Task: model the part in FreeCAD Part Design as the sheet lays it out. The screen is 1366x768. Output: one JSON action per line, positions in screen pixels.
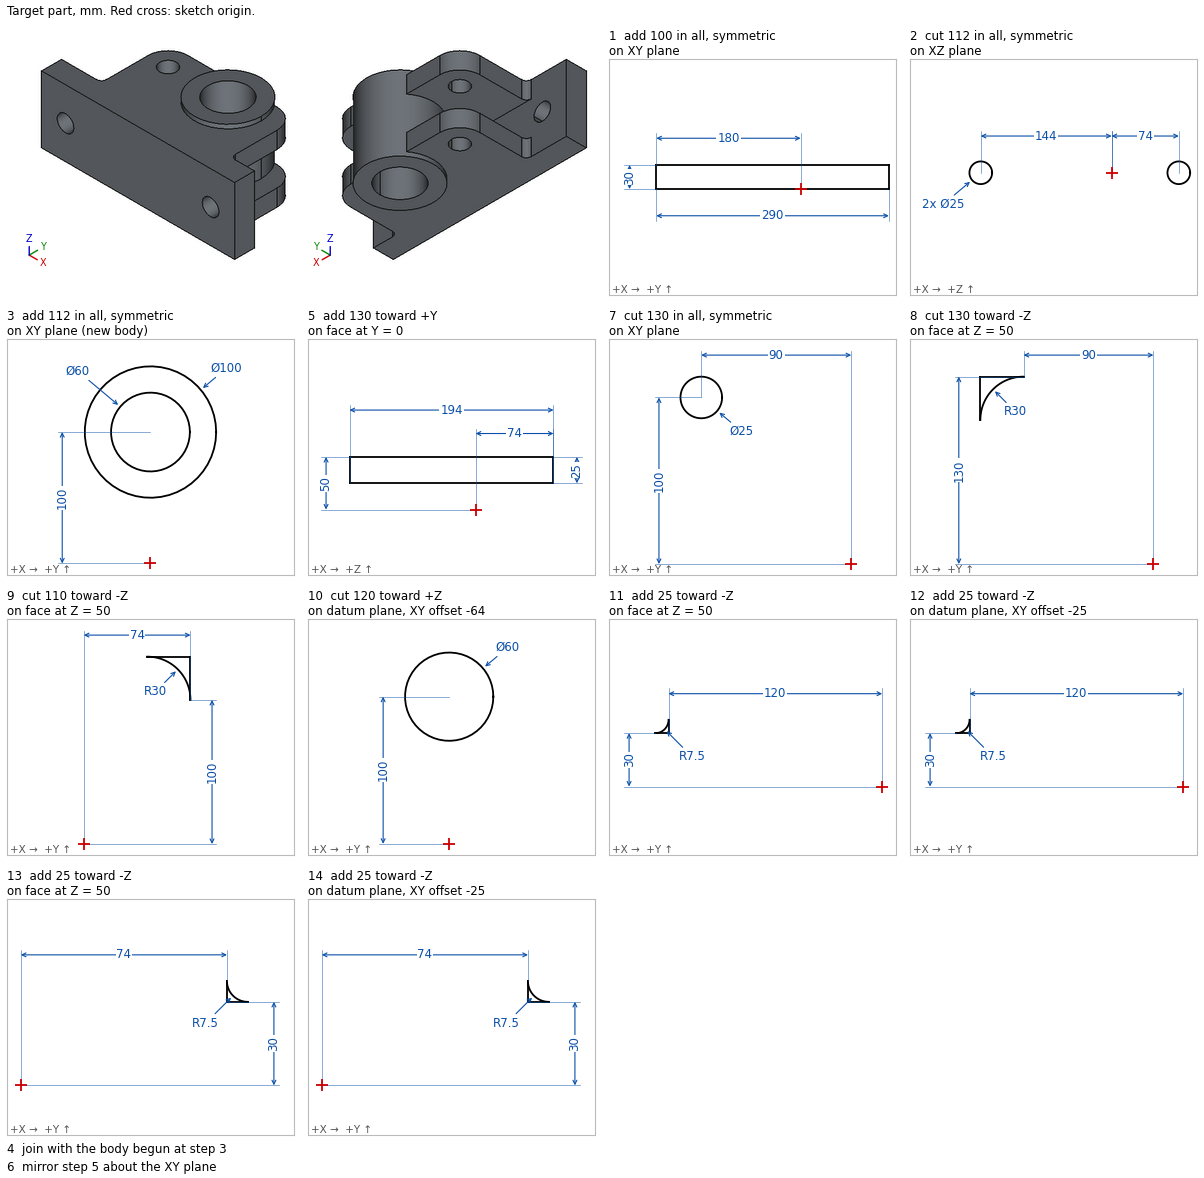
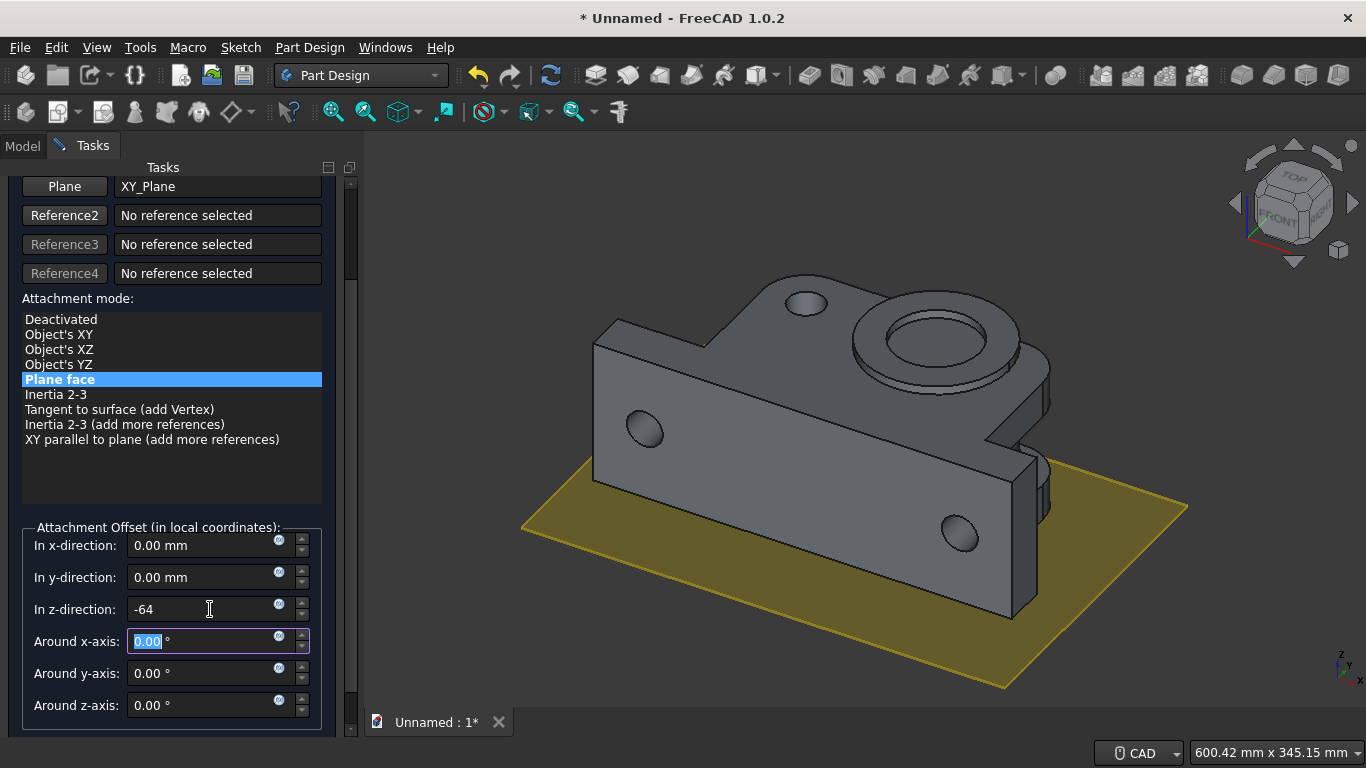
{"action": "scroll", "coordinate": [351, 456], "scroll_direction": "up", "scroll_amount": 3}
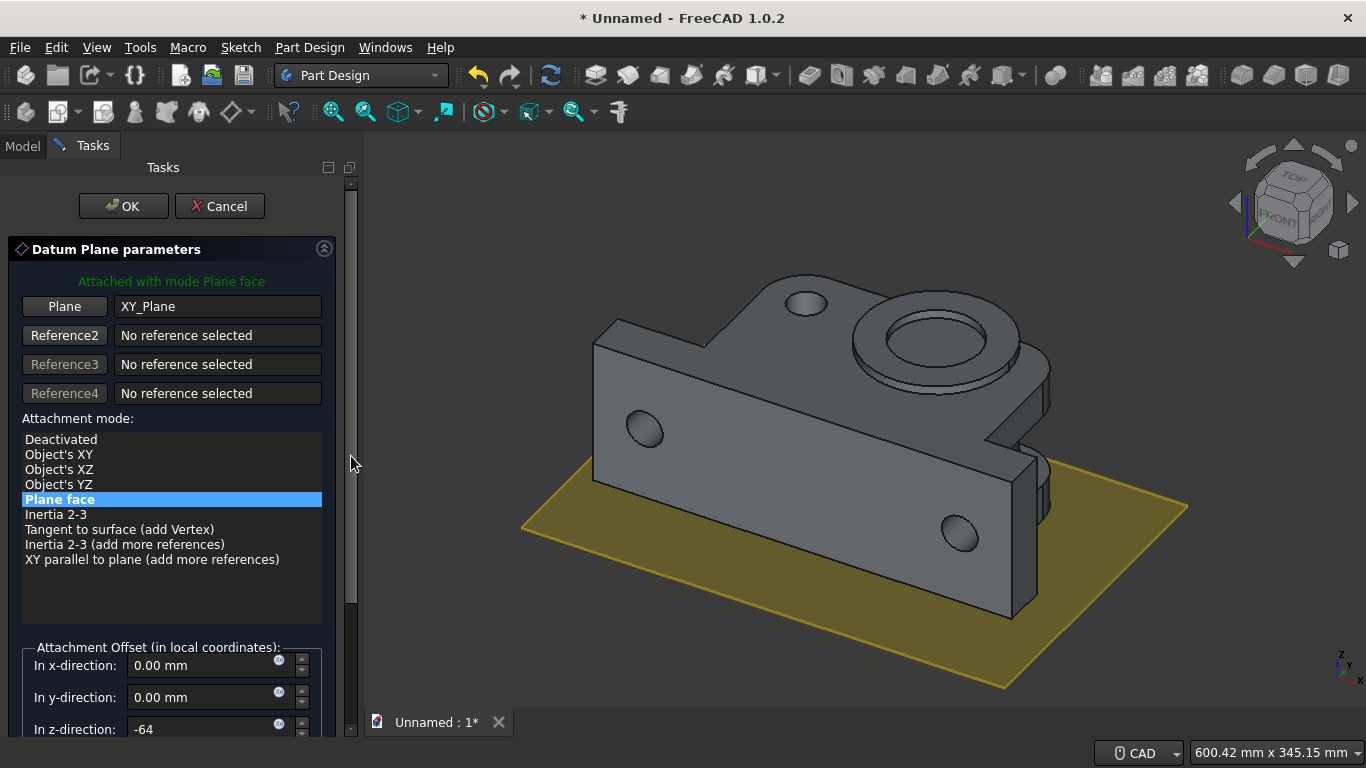
{"action": "left_click", "coordinate": [124, 206]}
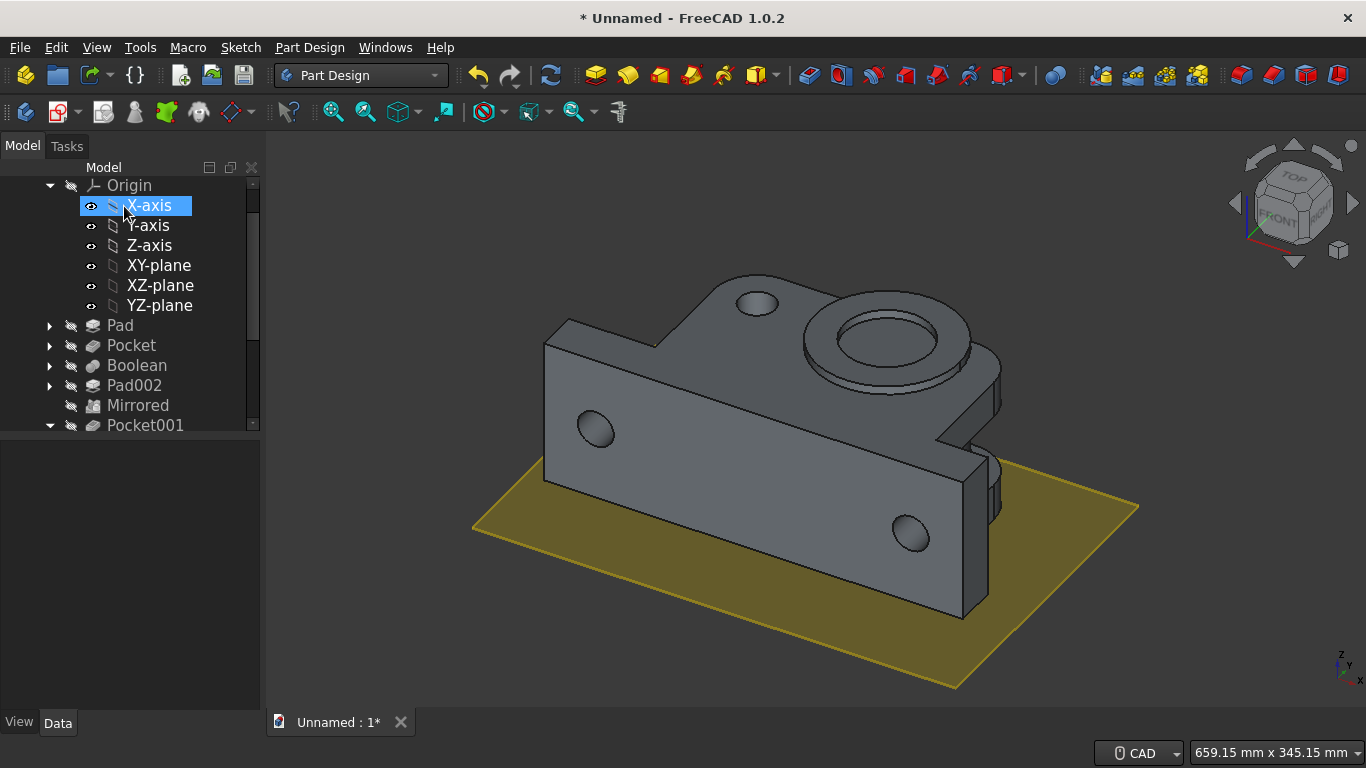
{"action": "scroll", "coordinate": [140, 301], "scroll_direction": "down", "scroll_amount": 3}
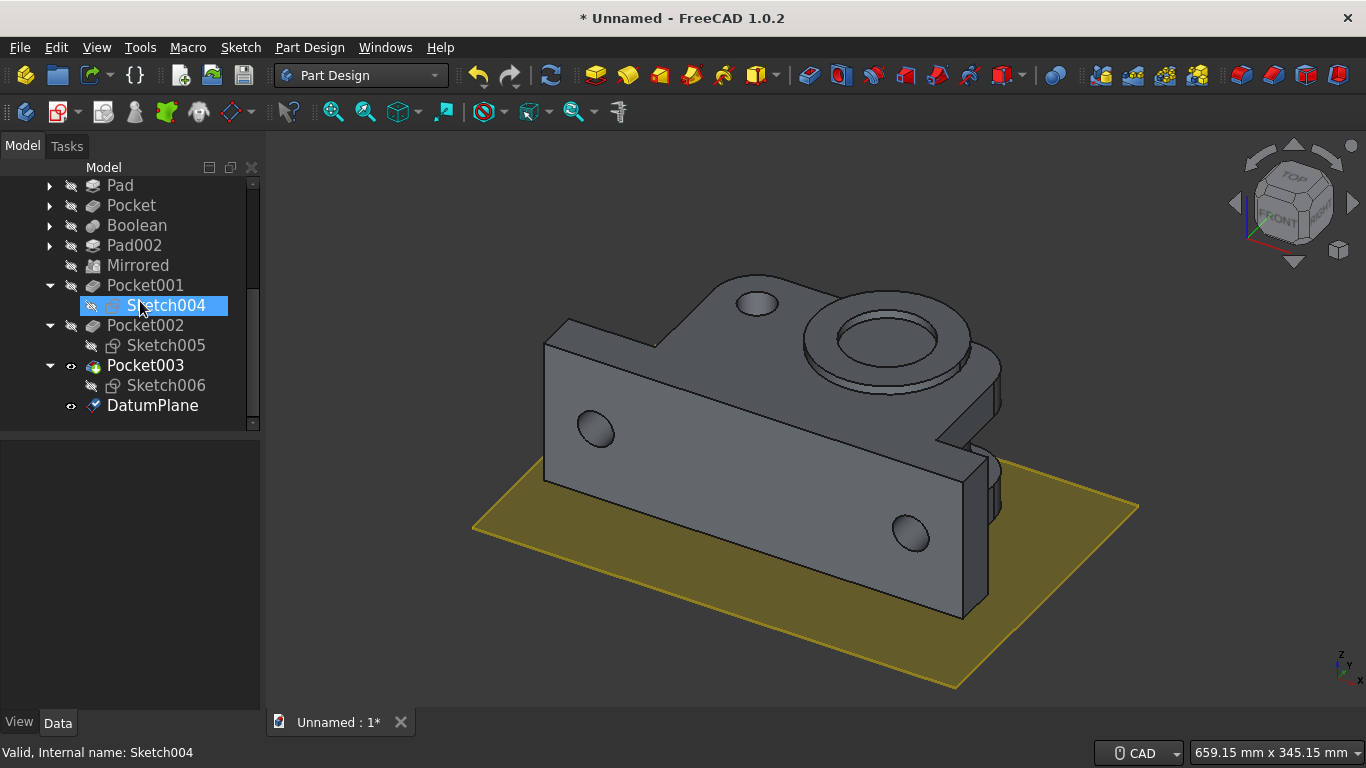
{"action": "left_click", "coordinate": [116, 406]}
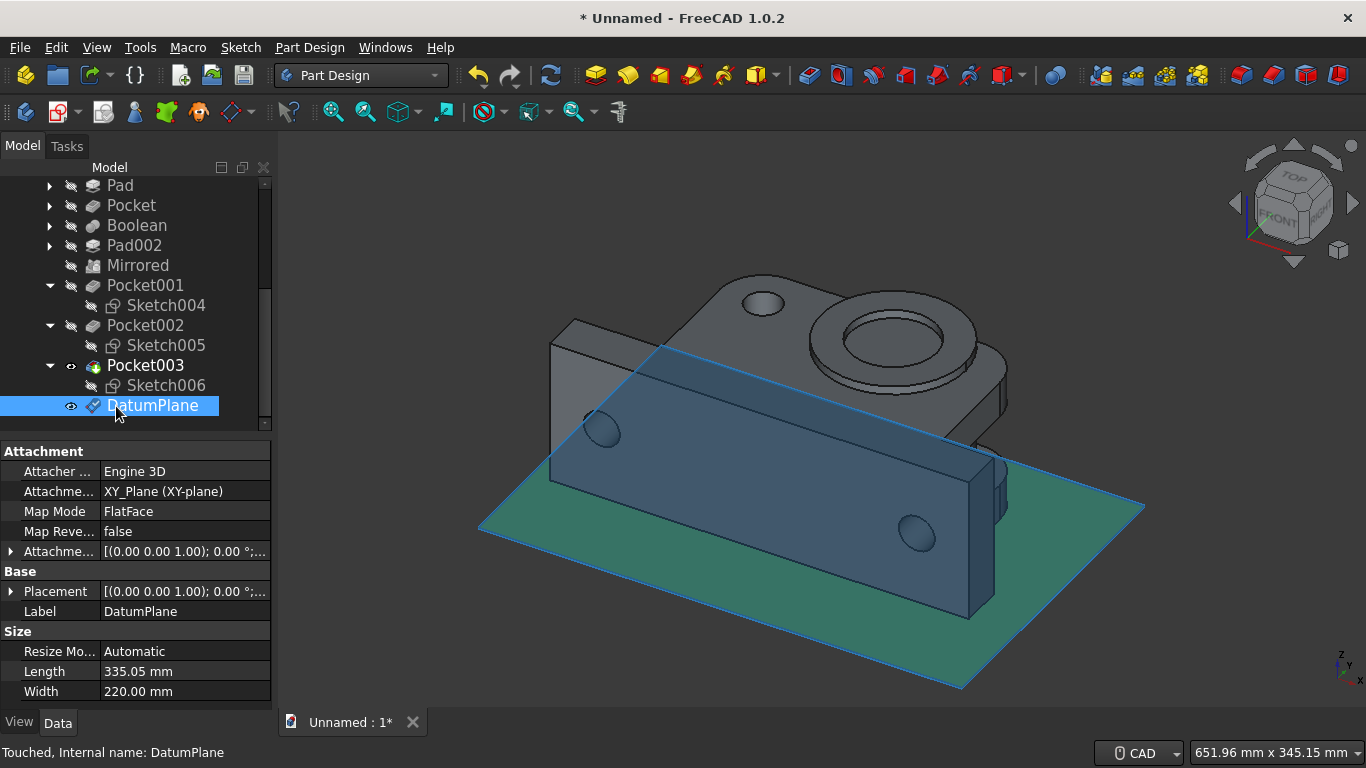
{"action": "left_click", "coordinate": [58, 112]}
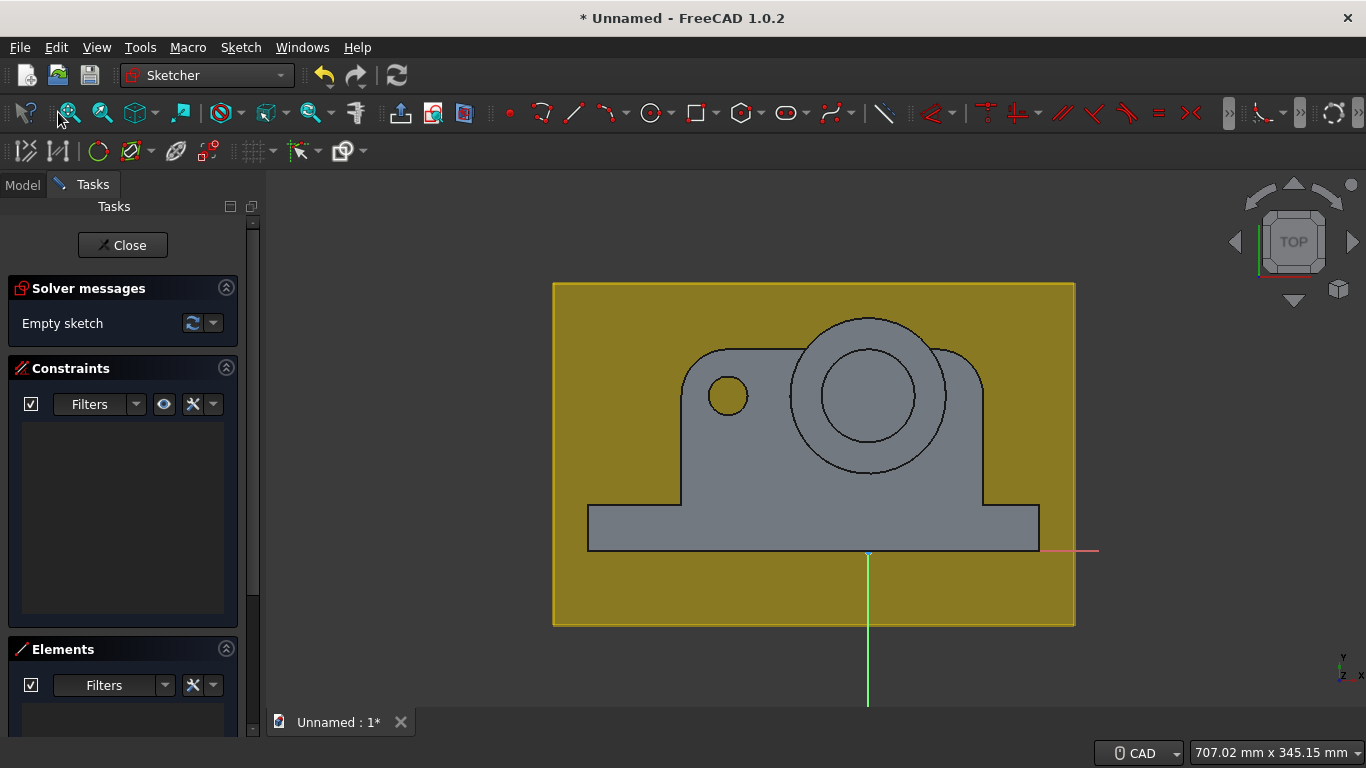
{"action": "left_click", "coordinate": [466, 114]}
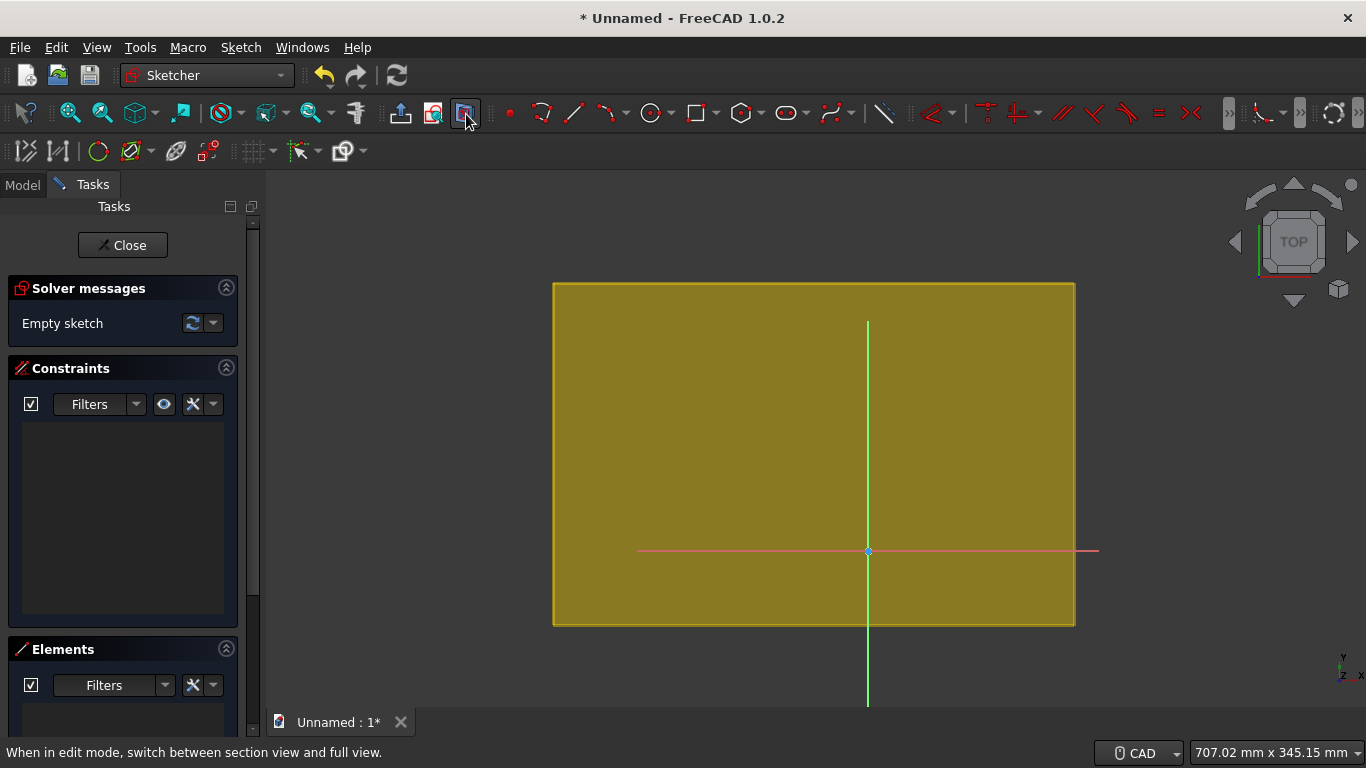
{"action": "scroll", "coordinate": [1015, 465], "scroll_direction": "up", "scroll_amount": 3}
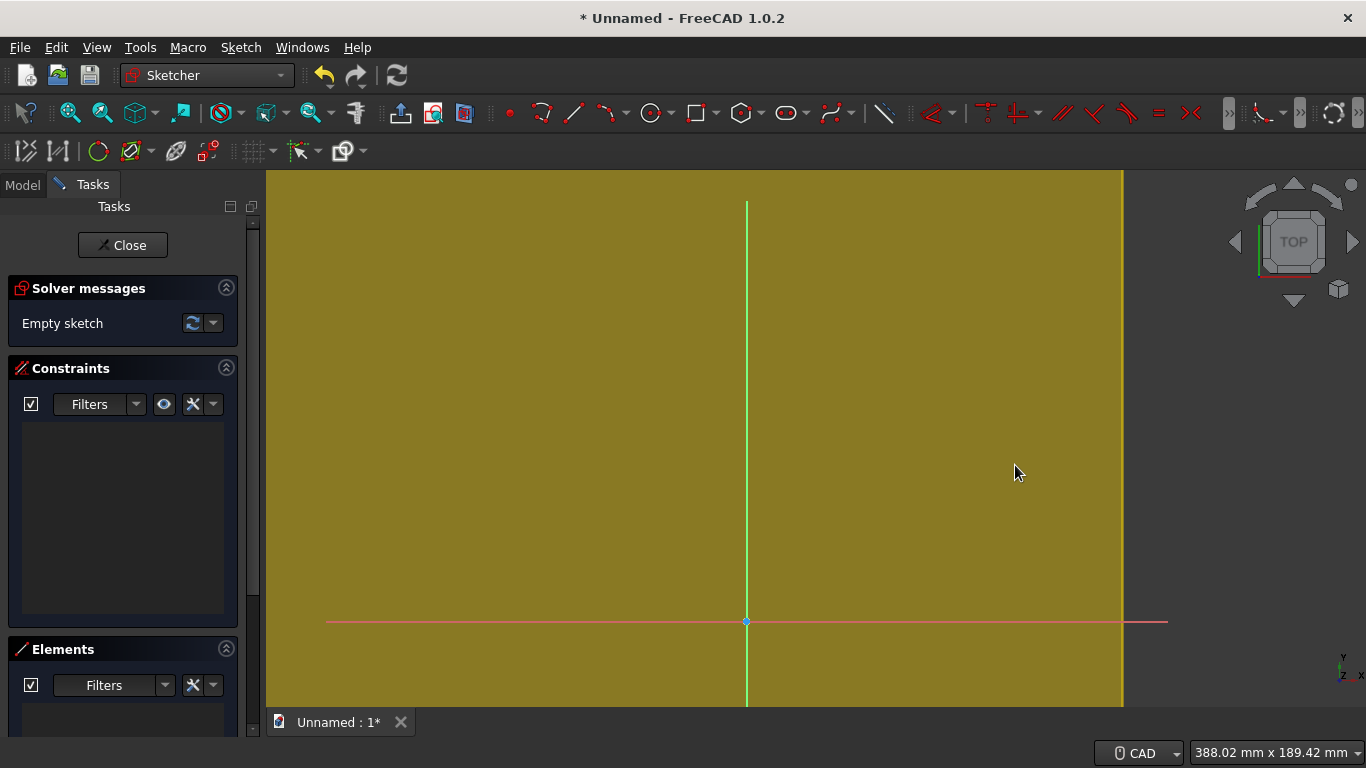
{"action": "left_click", "coordinate": [652, 114]}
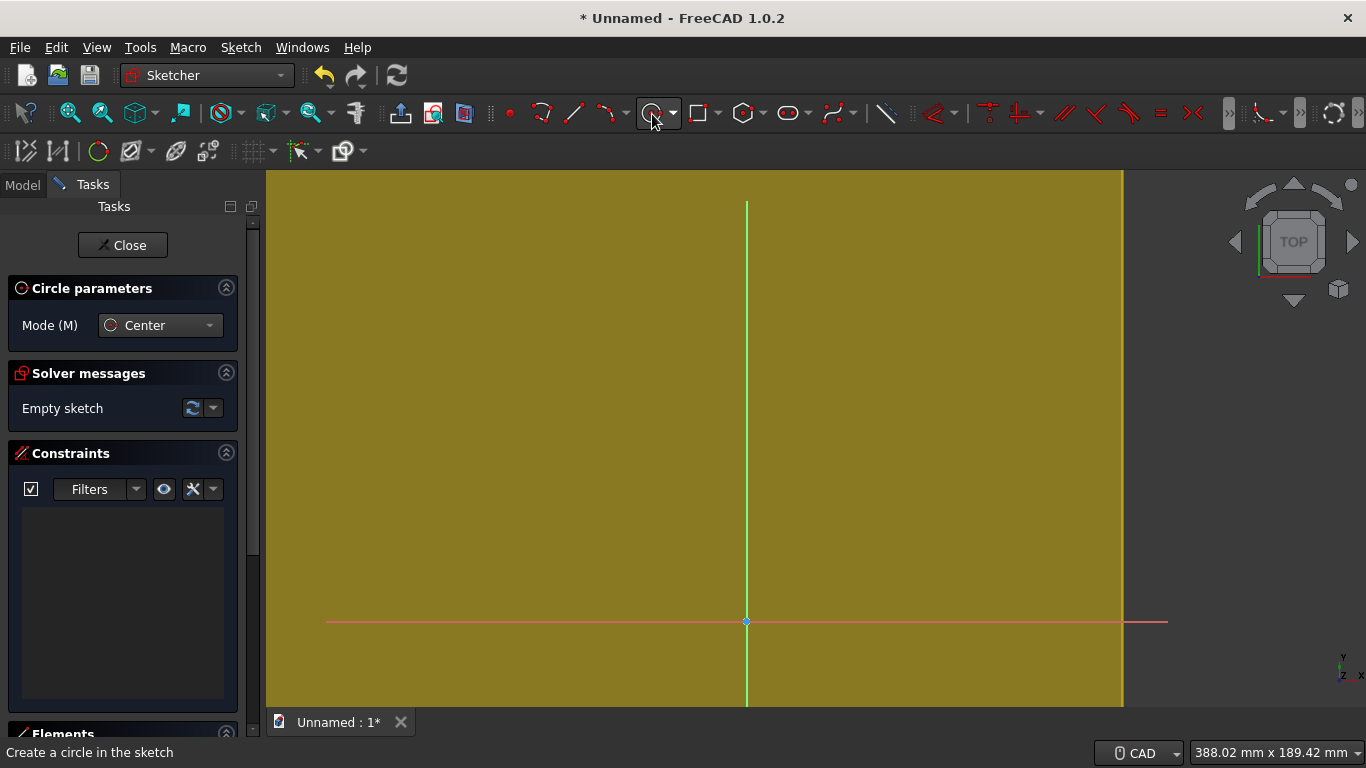
{"action": "left_click", "coordinate": [747, 339]}
{"action": "mouse_move", "coordinate": [807, 278]}